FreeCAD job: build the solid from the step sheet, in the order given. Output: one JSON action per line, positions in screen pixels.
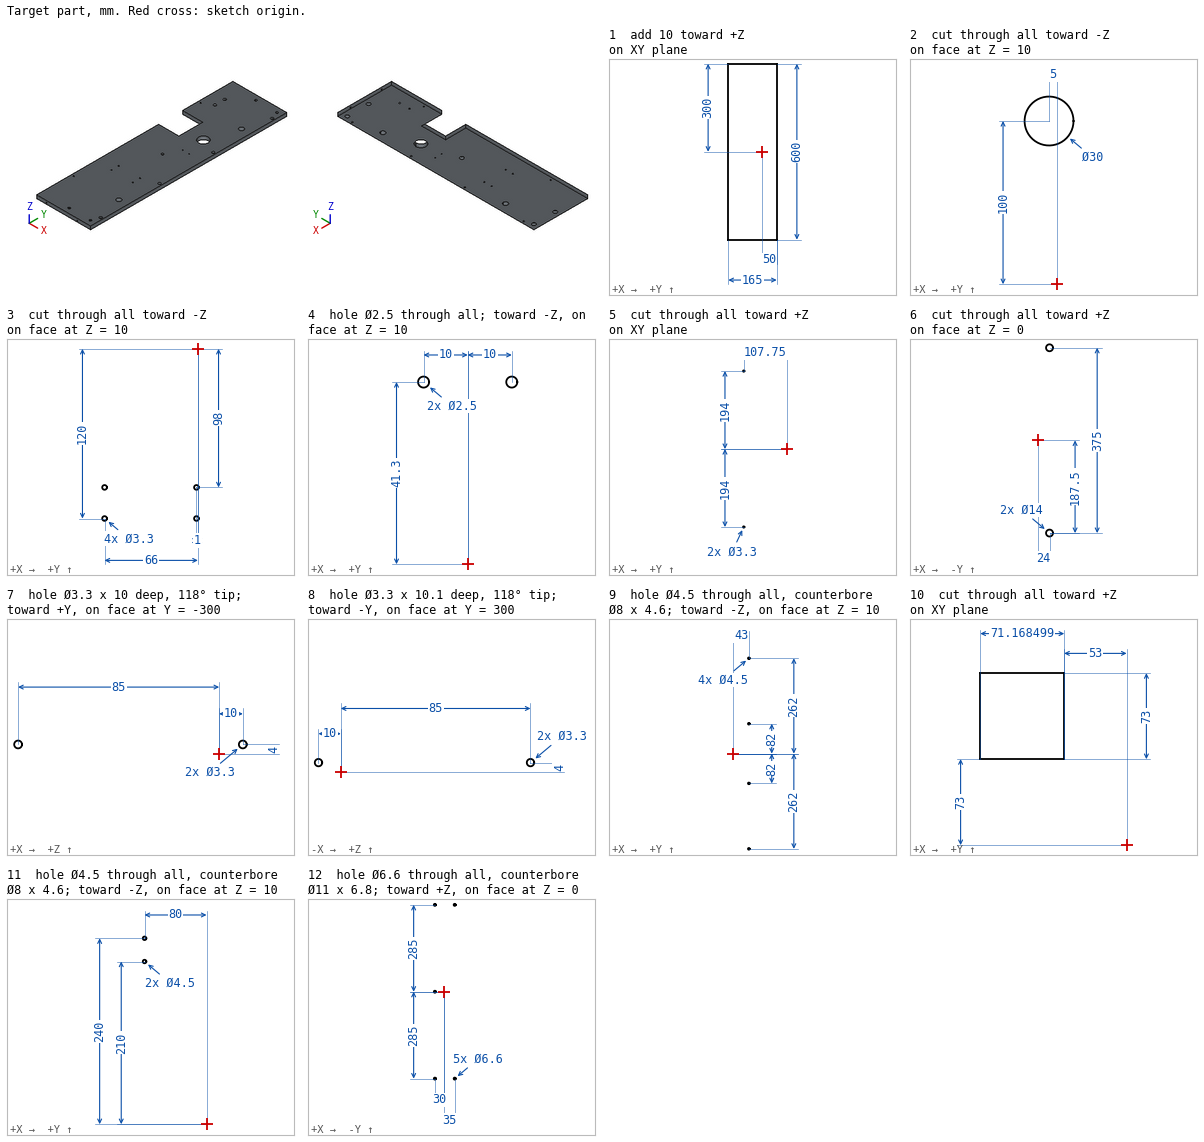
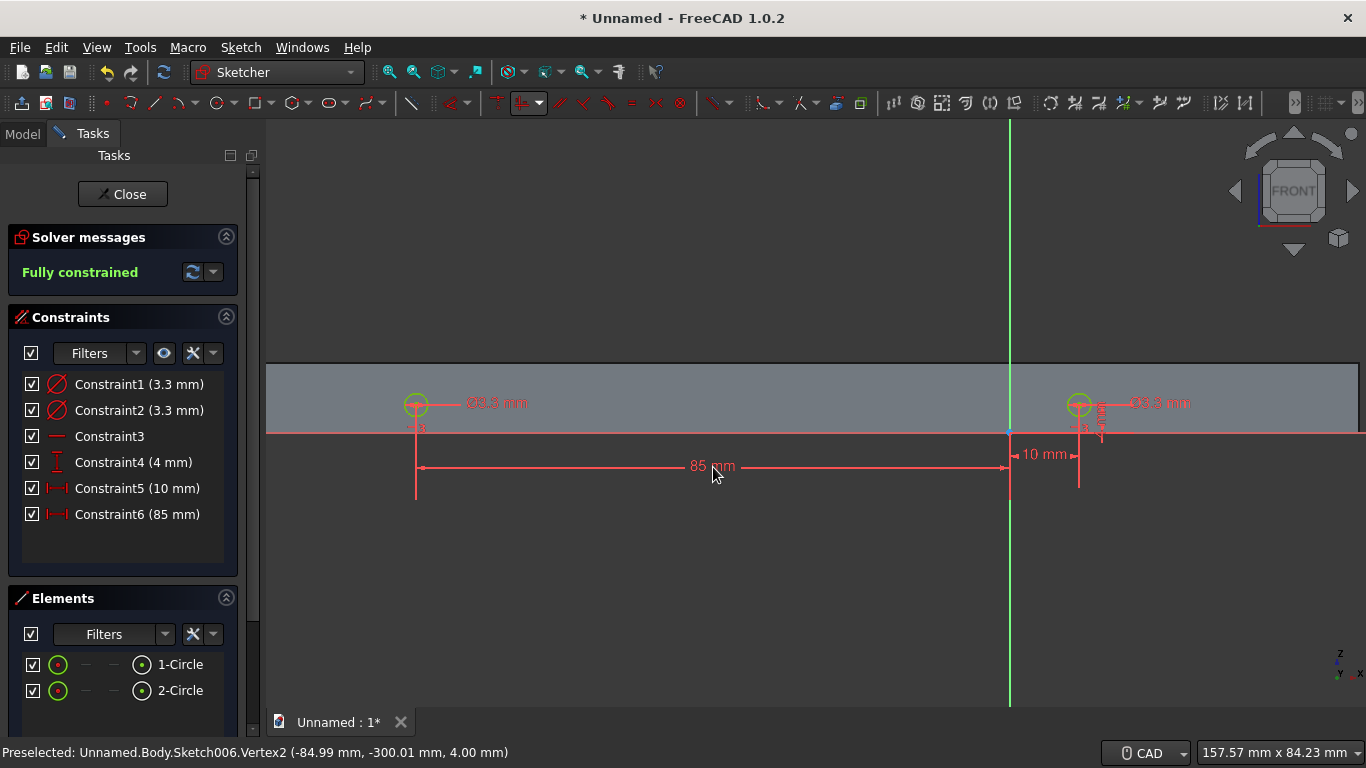
{"action": "left_click", "coordinate": [123, 194]}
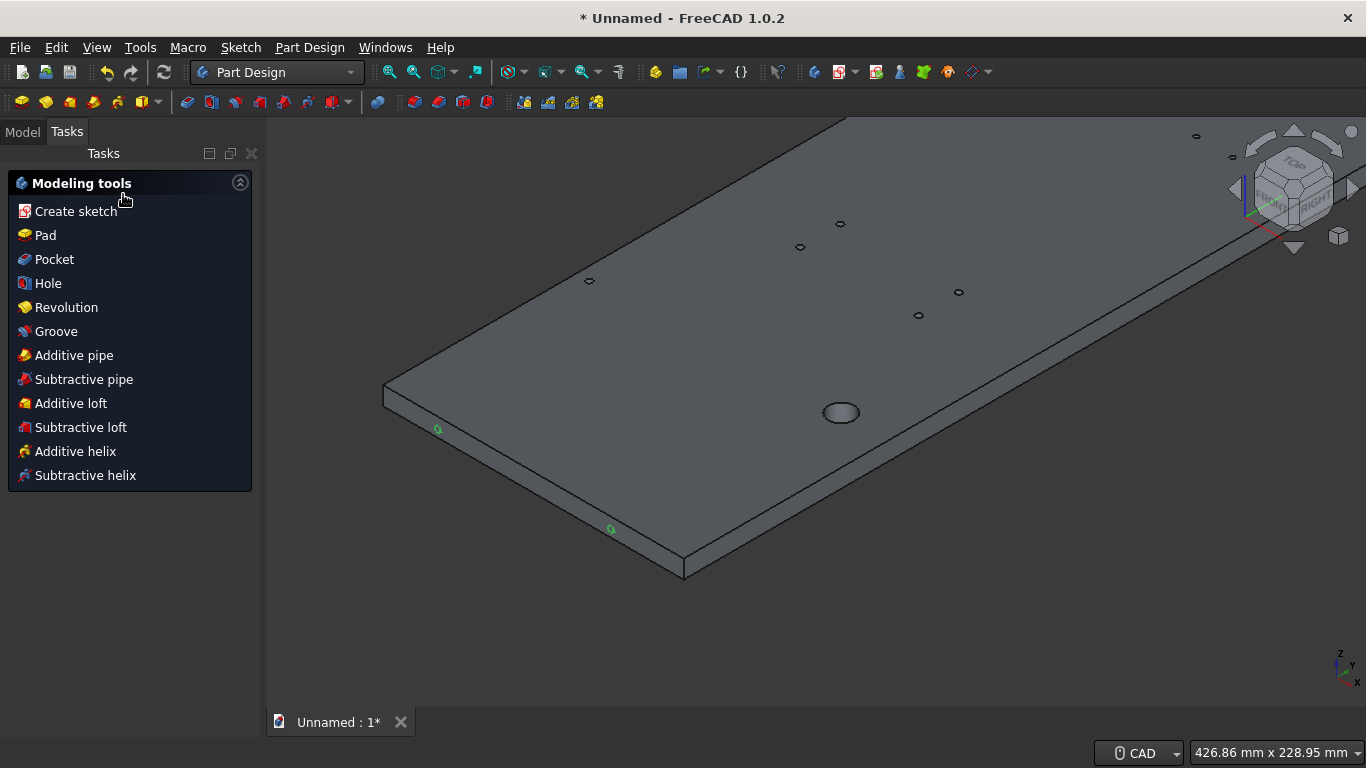
{"action": "left_click", "coordinate": [212, 102]}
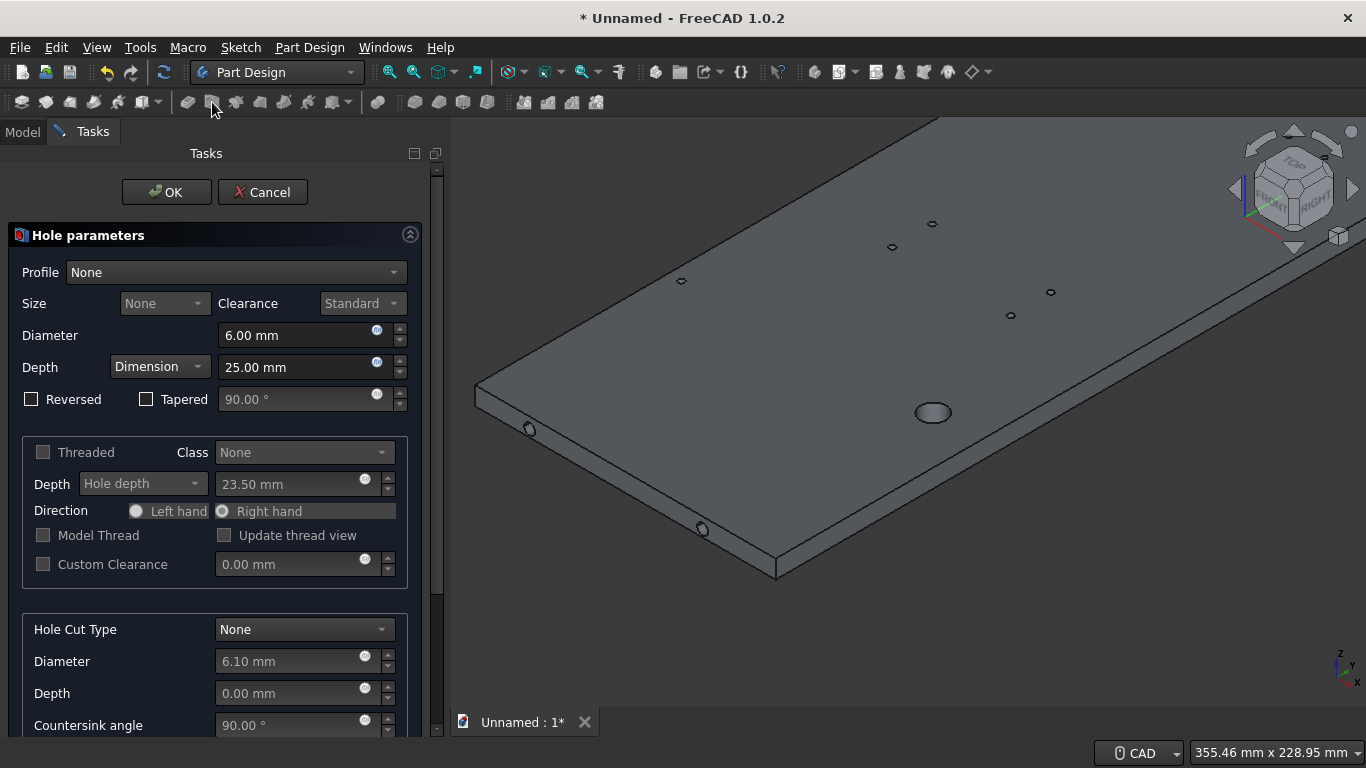
{"action": "triple_click", "coordinate": [305, 335]}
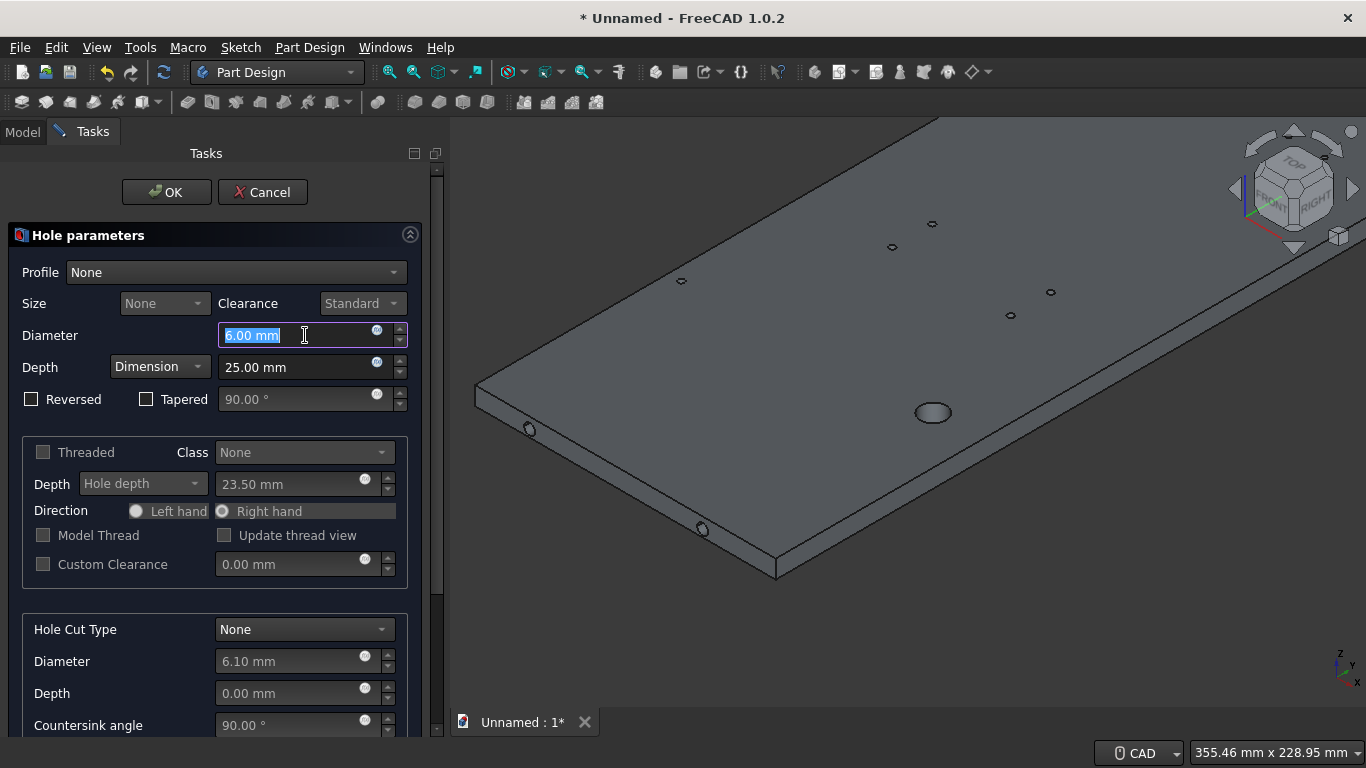
{"action": "type", "text": "3.3"}
{"action": "key", "text": "Tab"}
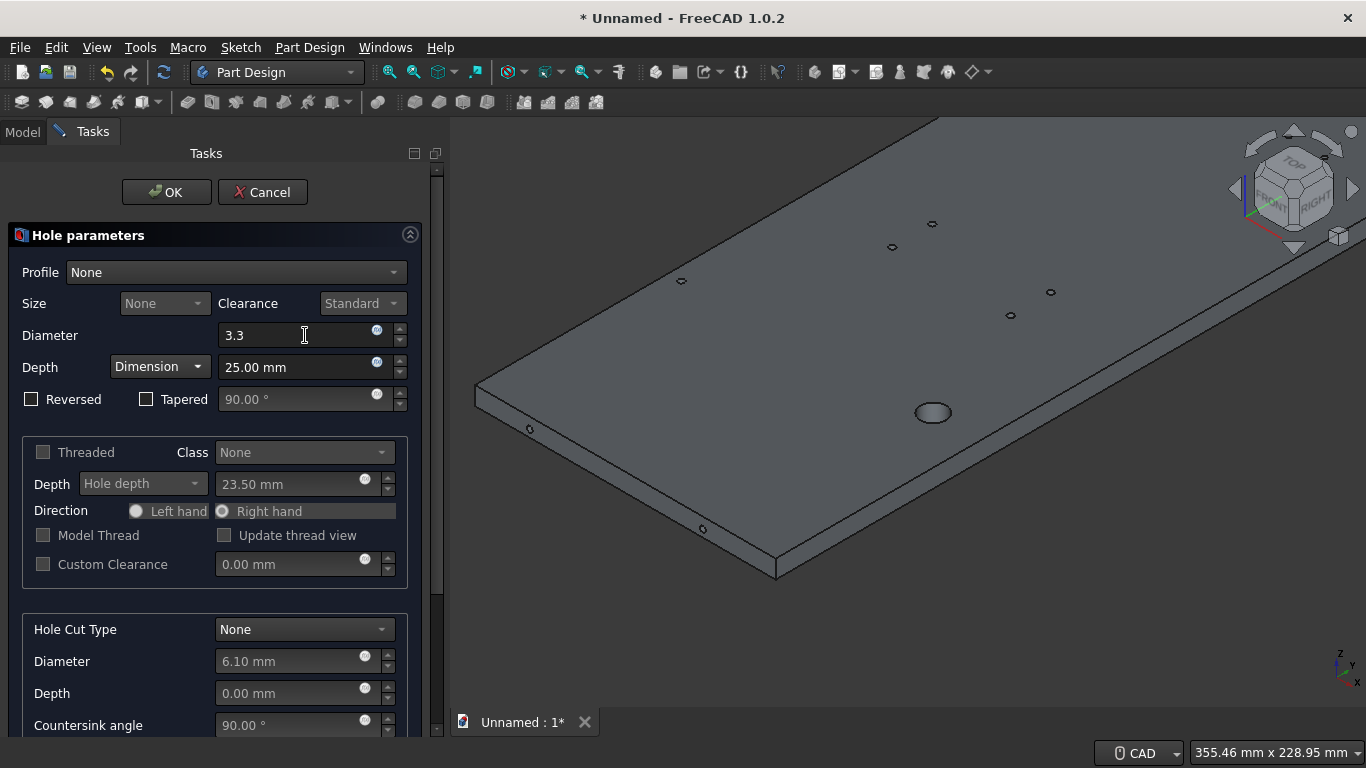
{"action": "triple_click", "coordinate": [305, 367]}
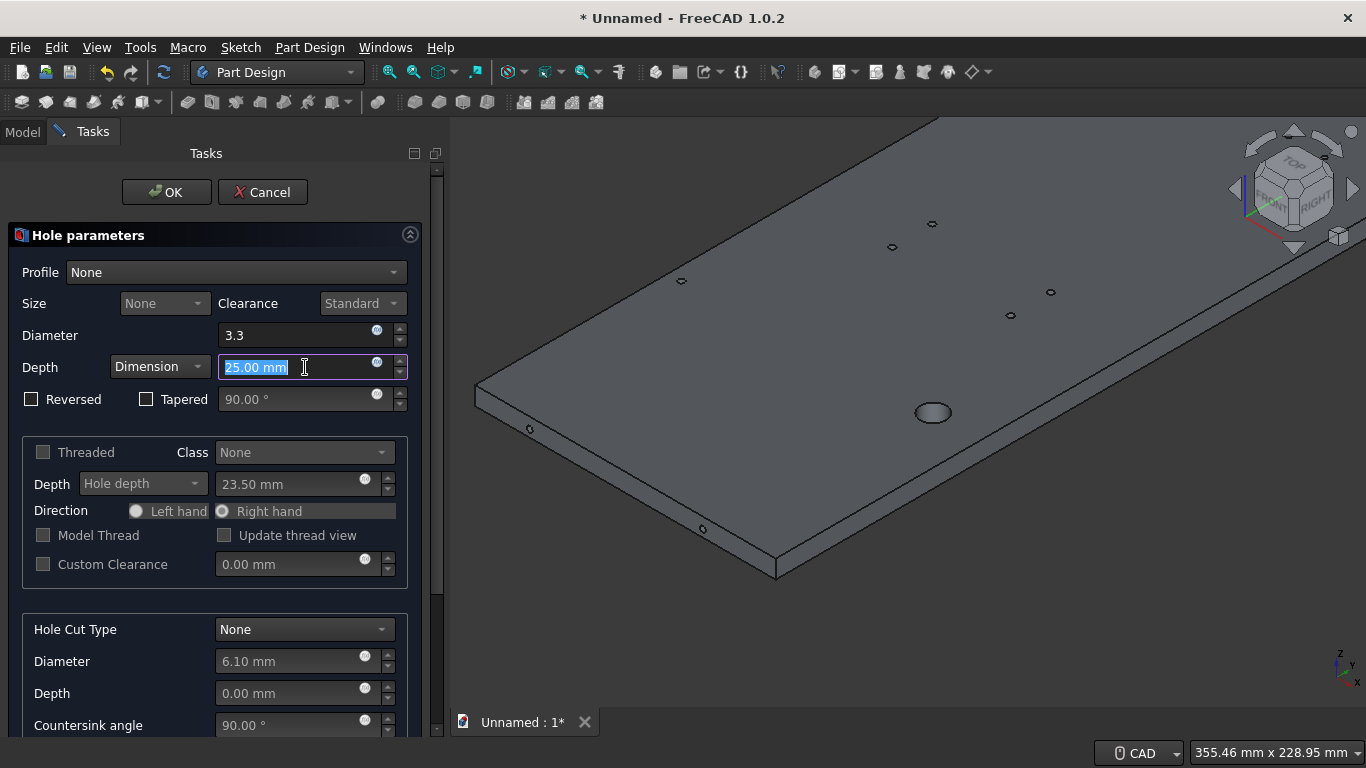
{"action": "type", "text": "10"}
{"action": "key", "text": "Tab"}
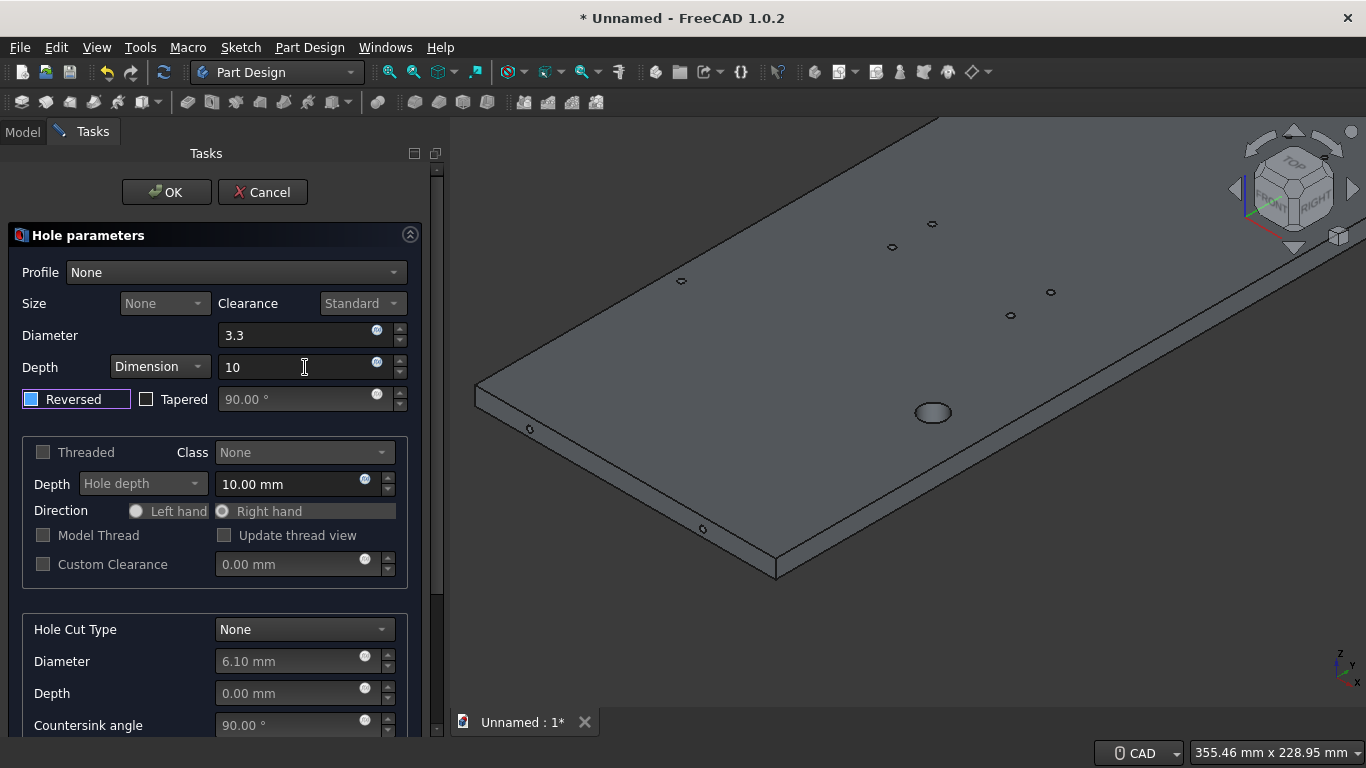
{"action": "left_click", "coordinate": [167, 192]}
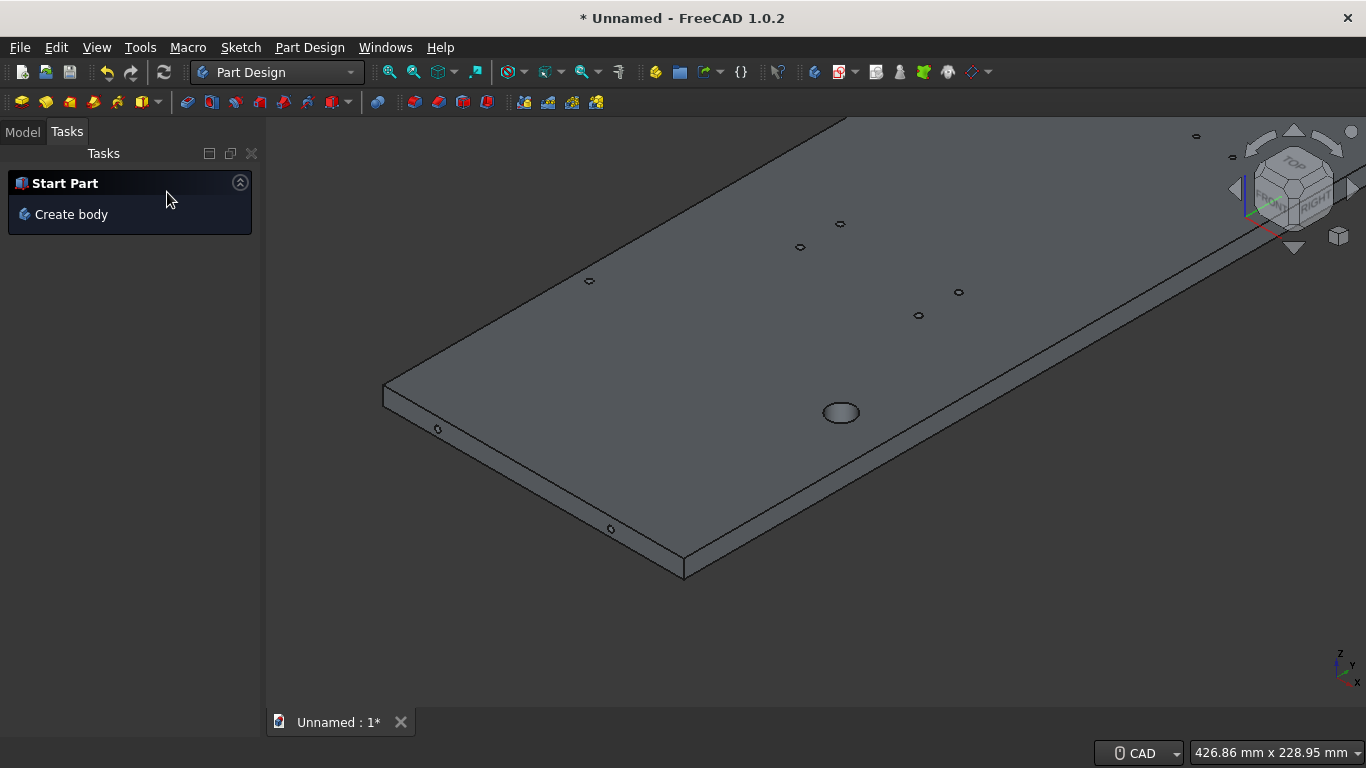
{"action": "left_click", "coordinate": [390, 72]}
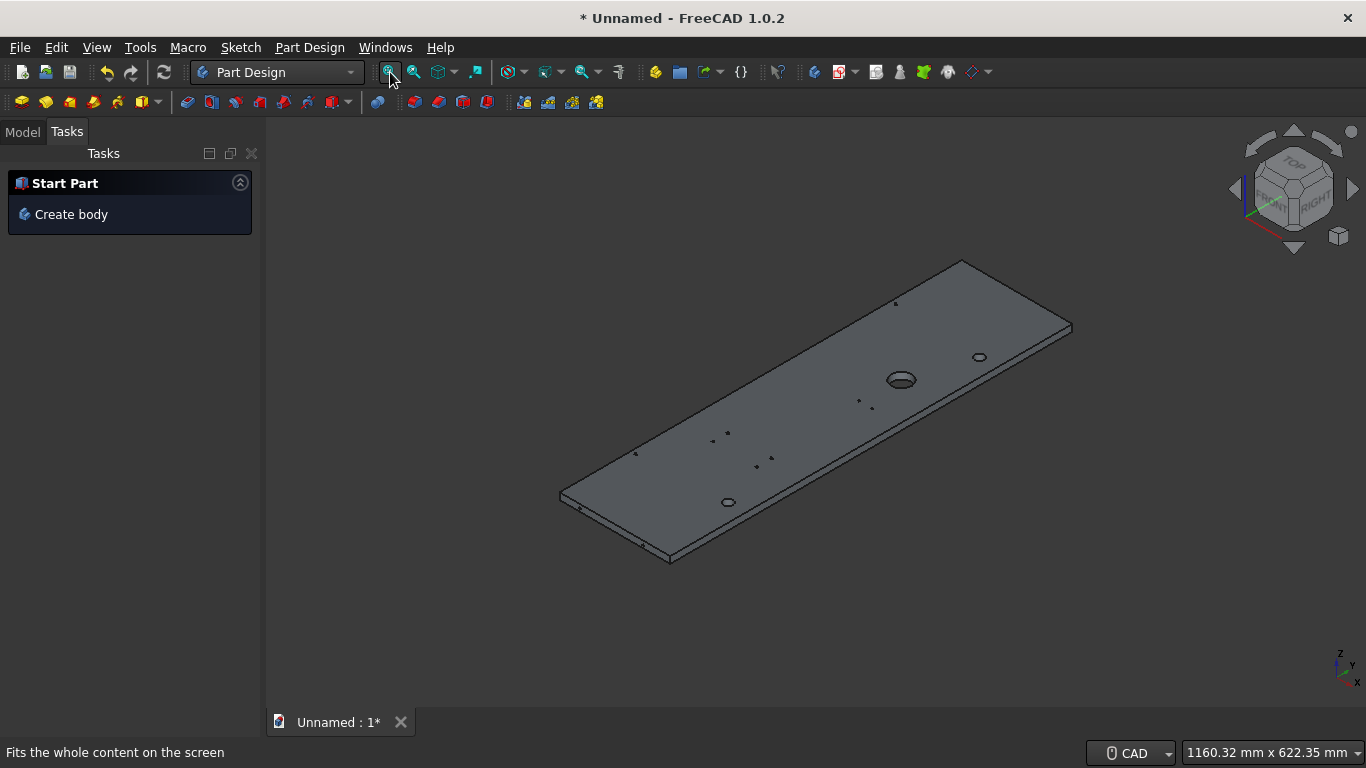
{"action": "key", "text": "4"}